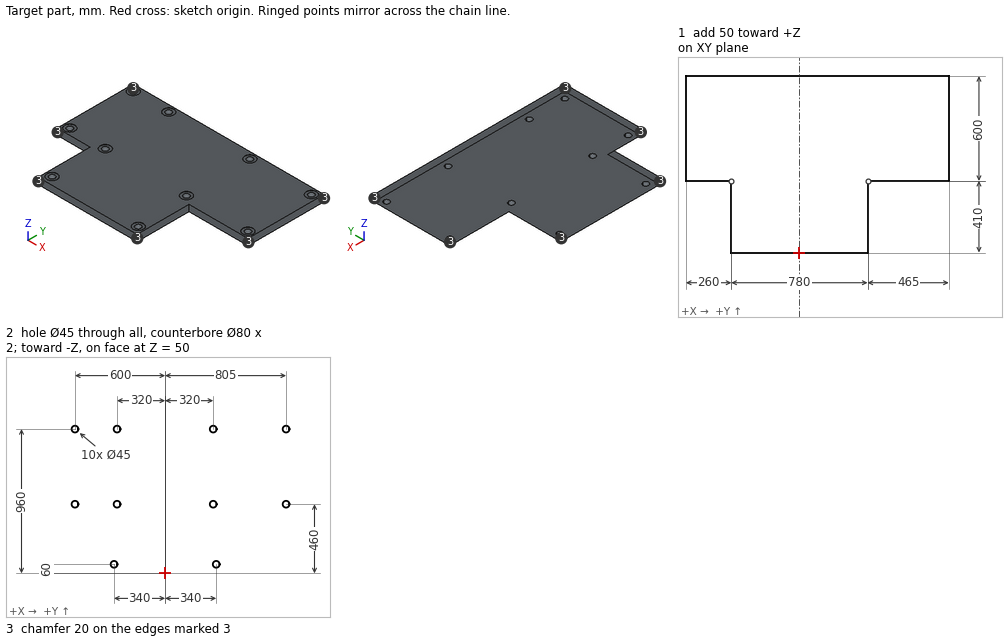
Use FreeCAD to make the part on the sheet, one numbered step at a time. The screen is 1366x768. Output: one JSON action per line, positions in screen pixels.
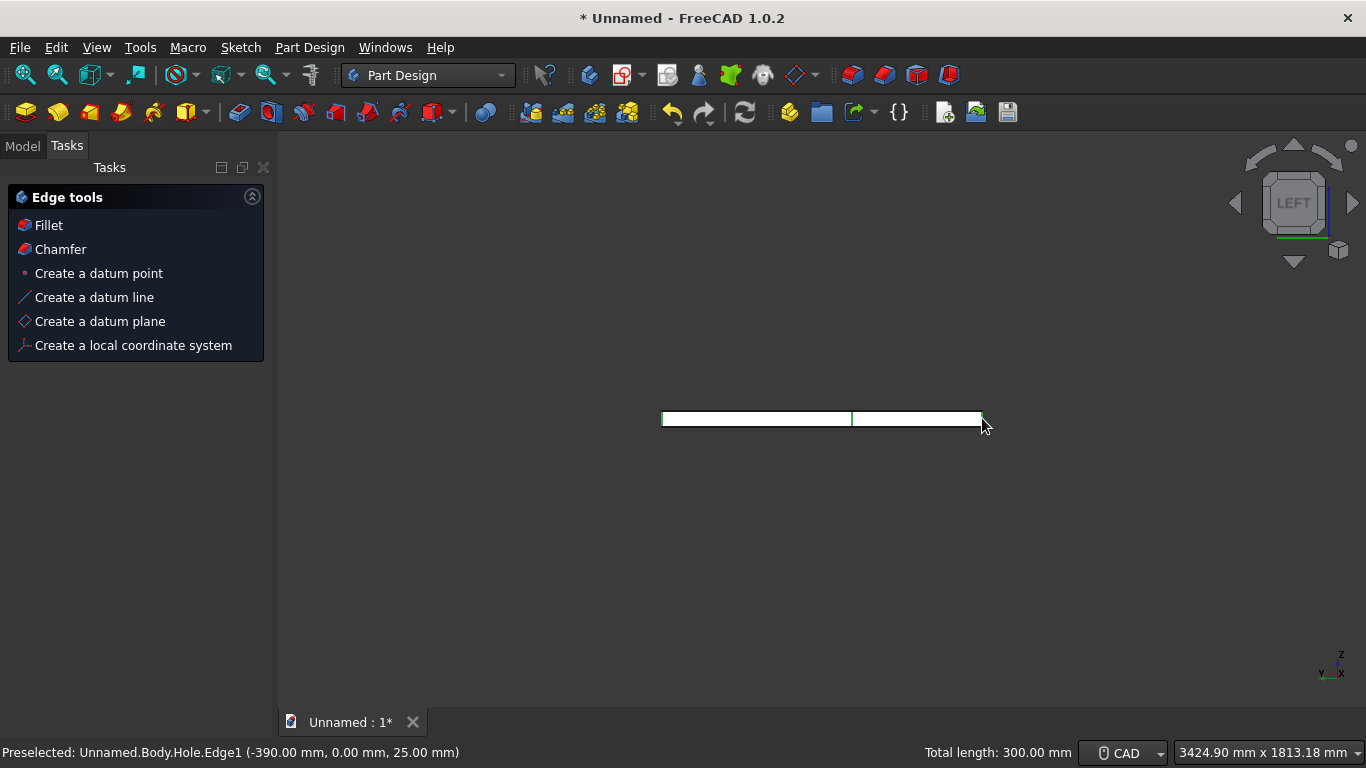
{"action": "left_click", "coordinate": [886, 76]}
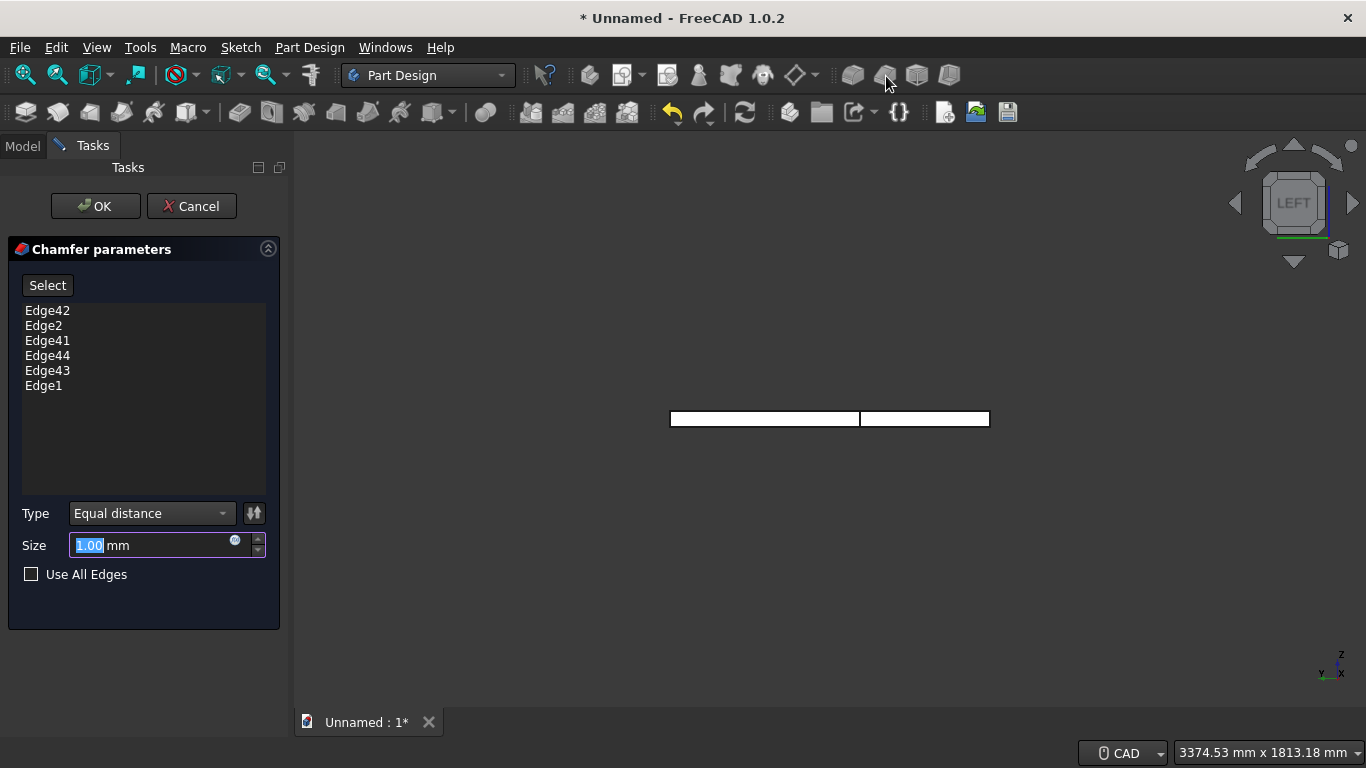
{"action": "type", "text": "20"}
{"action": "key", "text": "Tab"}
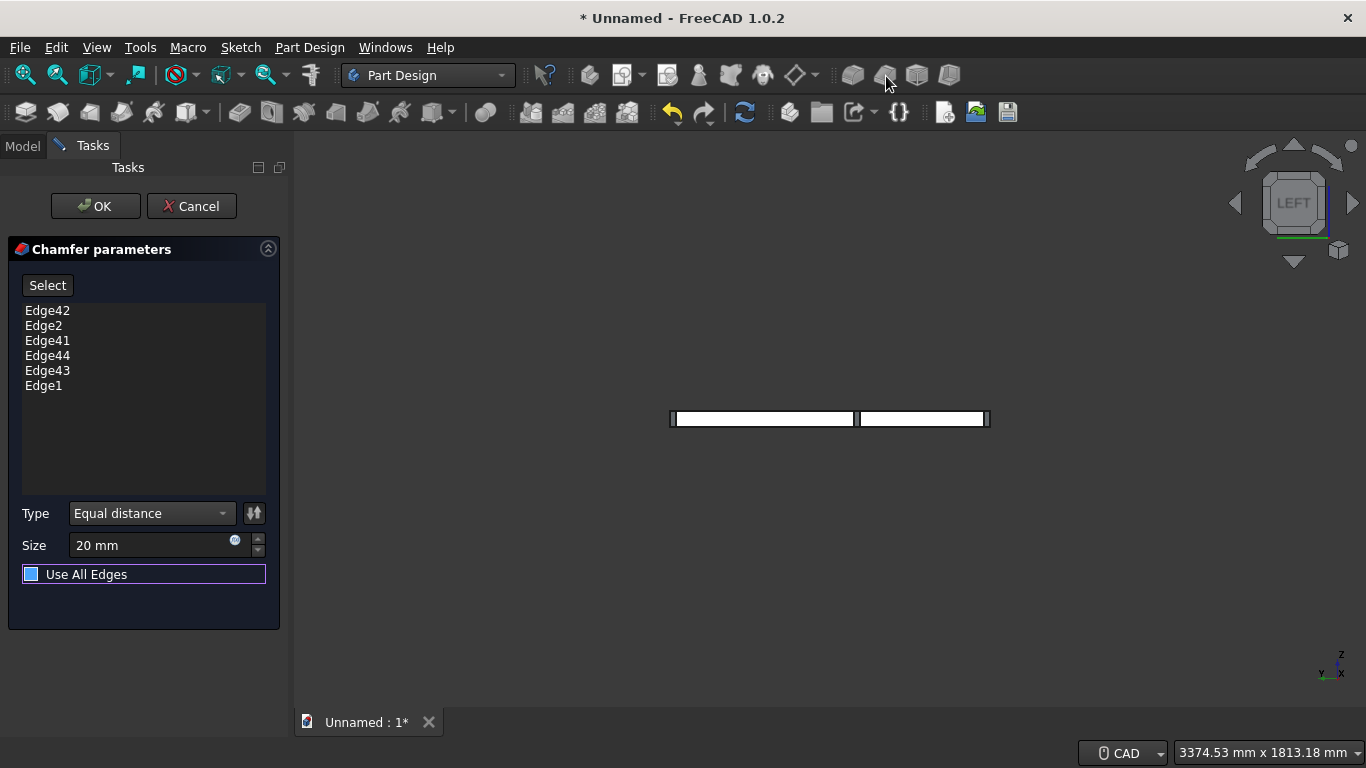
{"action": "left_click", "coordinate": [96, 206]}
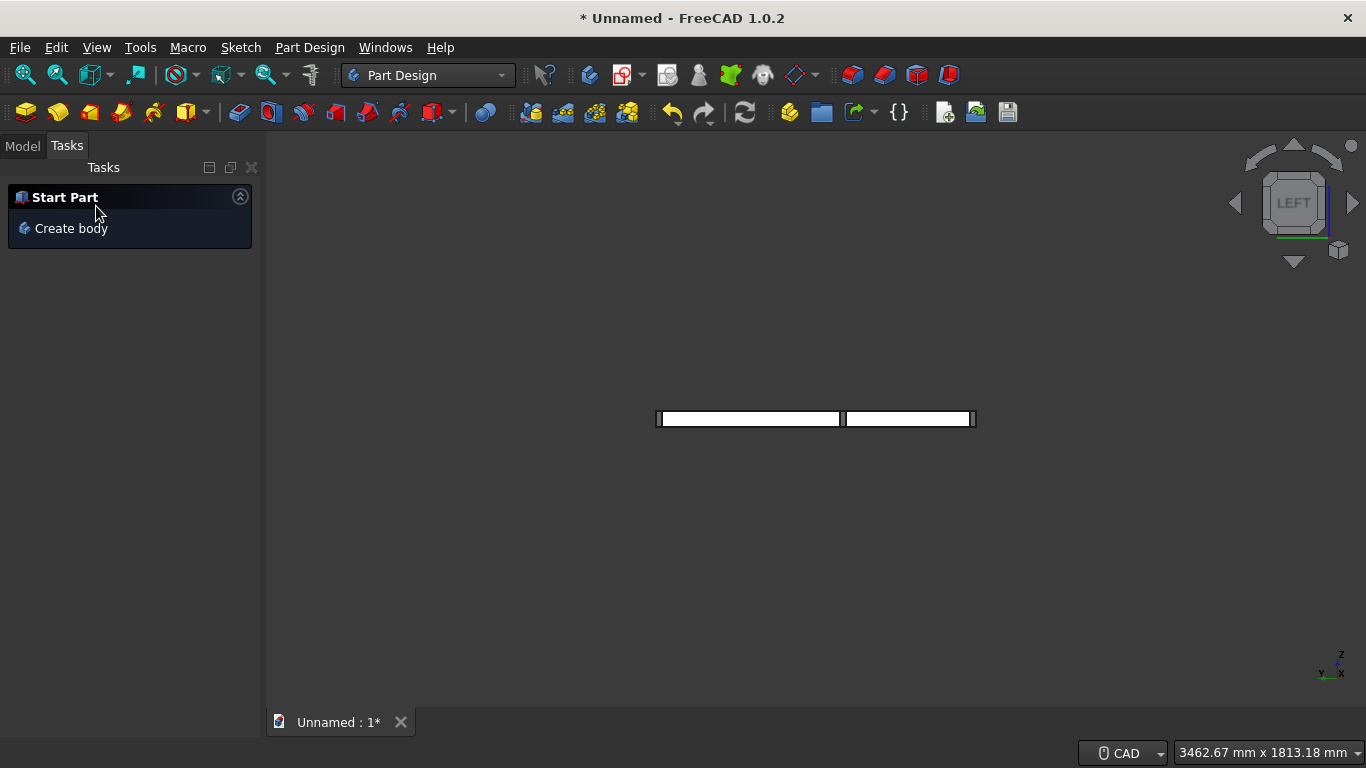
{"action": "key", "text": "0"}